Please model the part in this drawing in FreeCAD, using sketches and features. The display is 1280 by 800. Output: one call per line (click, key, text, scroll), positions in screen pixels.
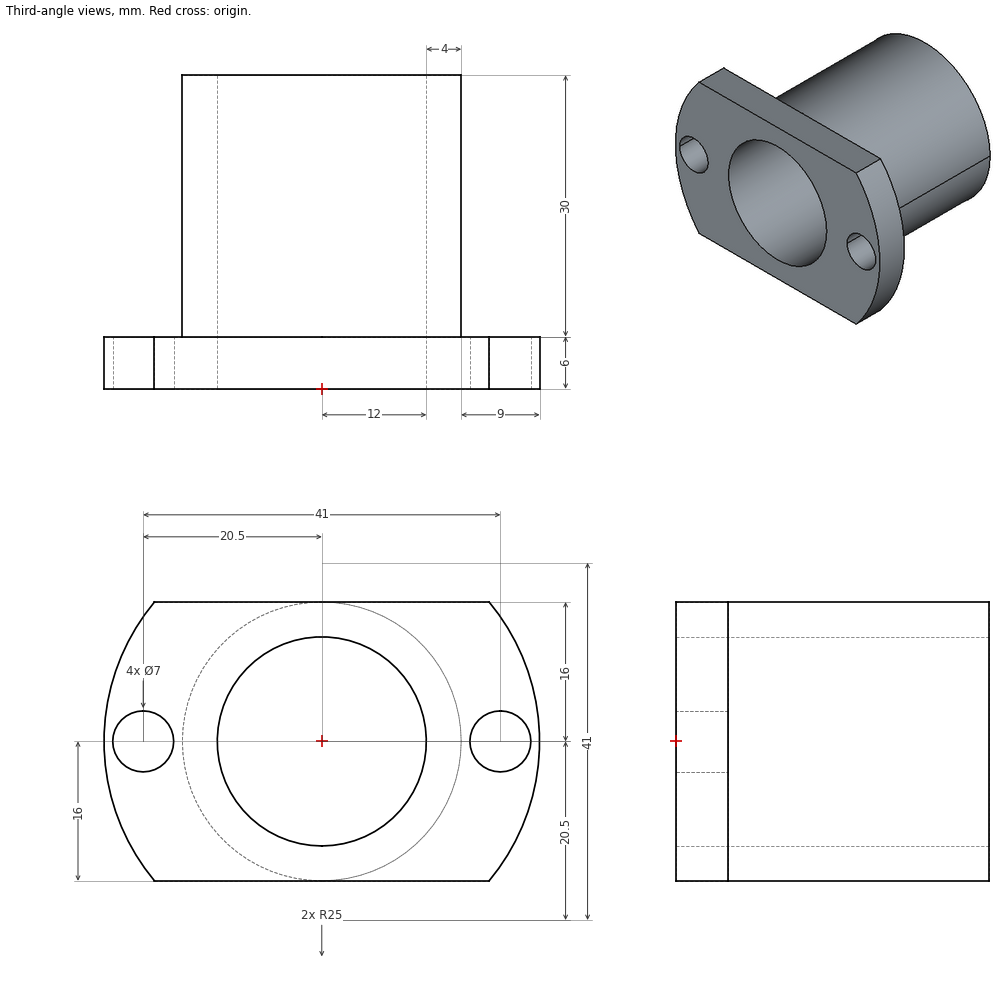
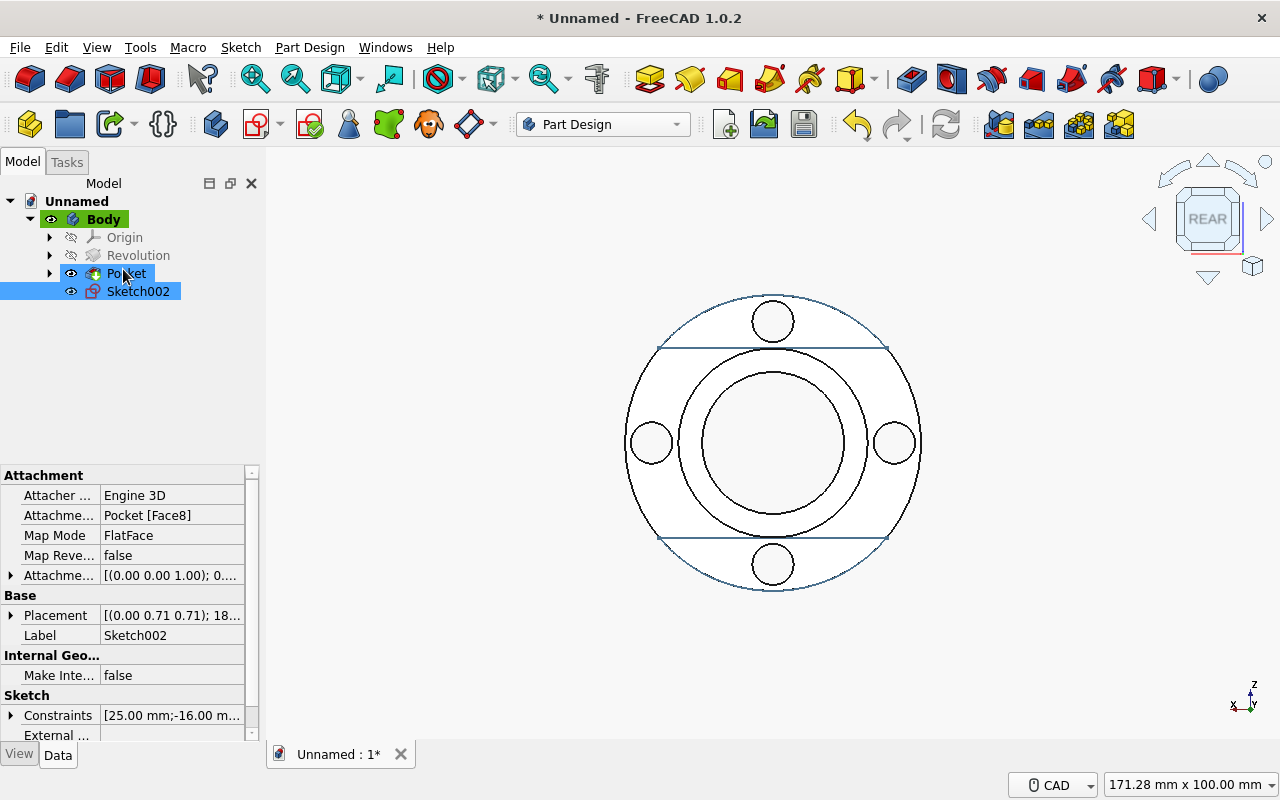
click(912, 80)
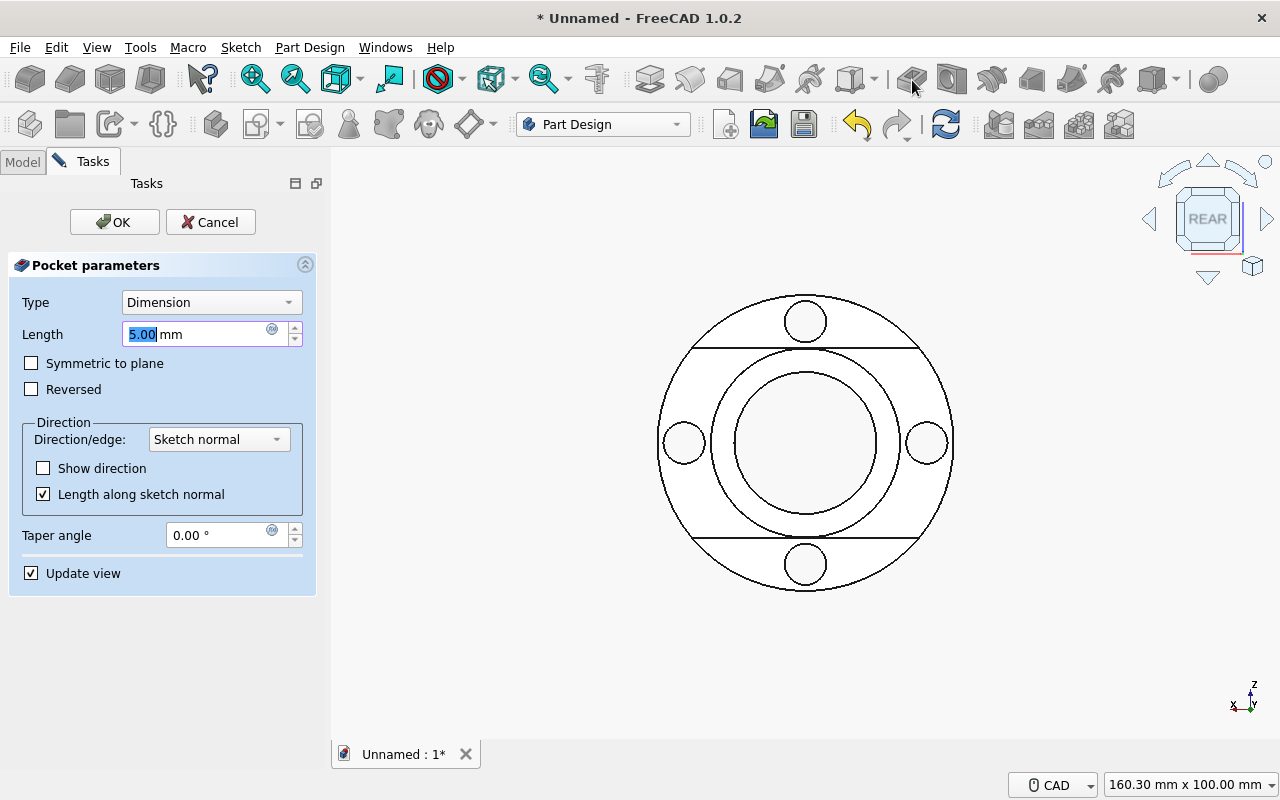
click(212, 302)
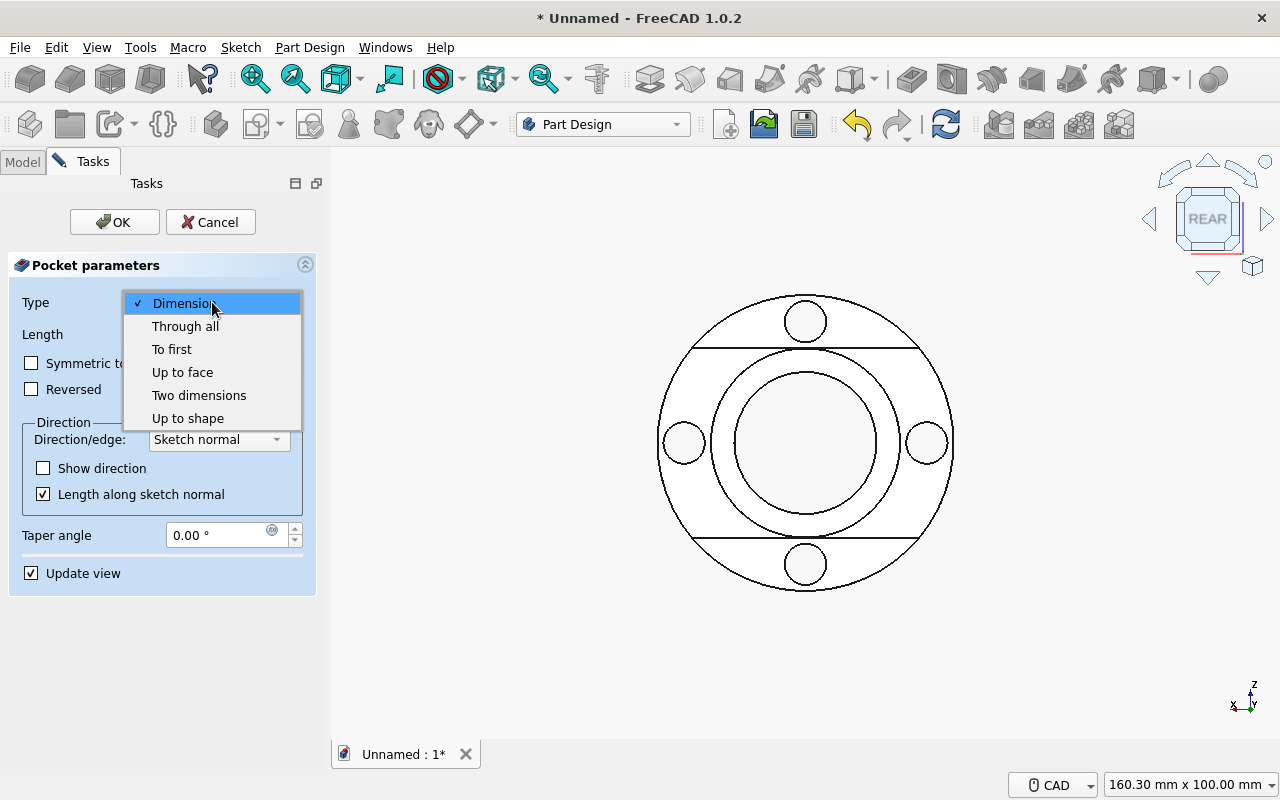
click(212, 326)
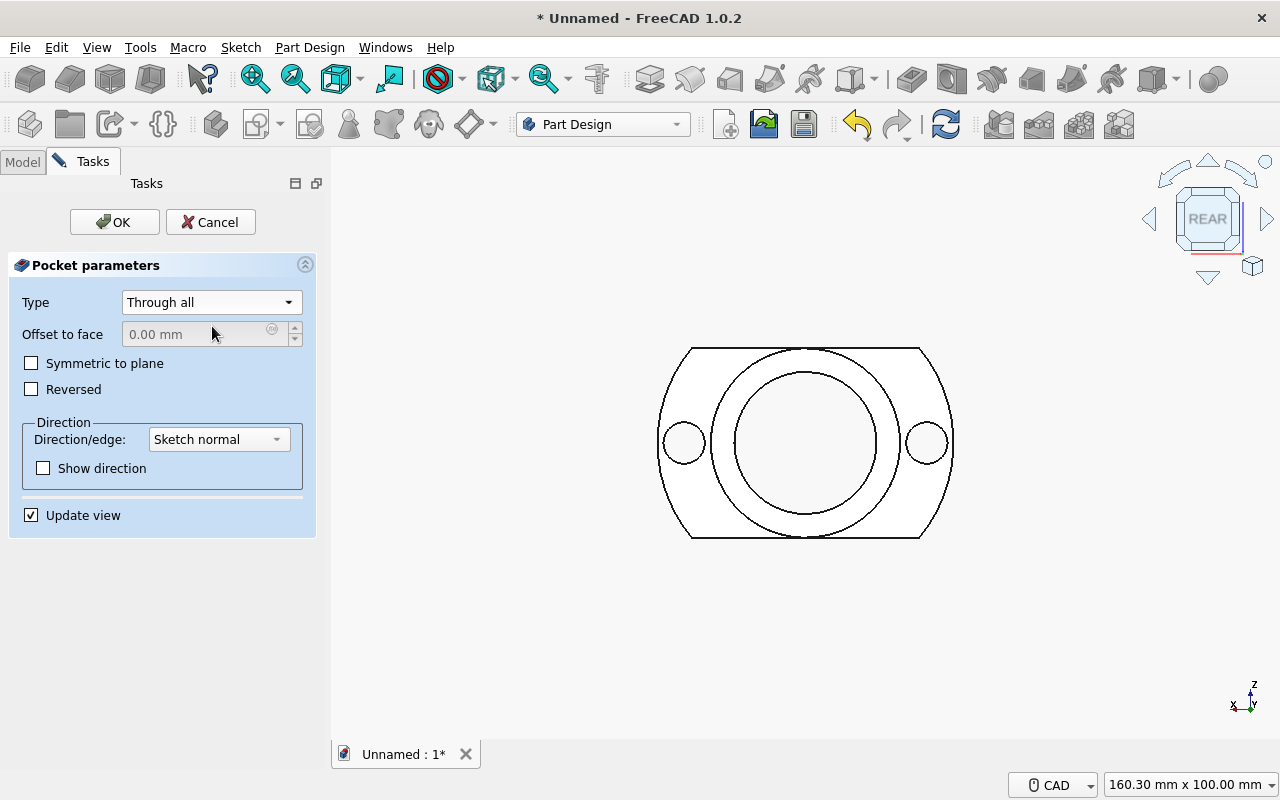
click(115, 222)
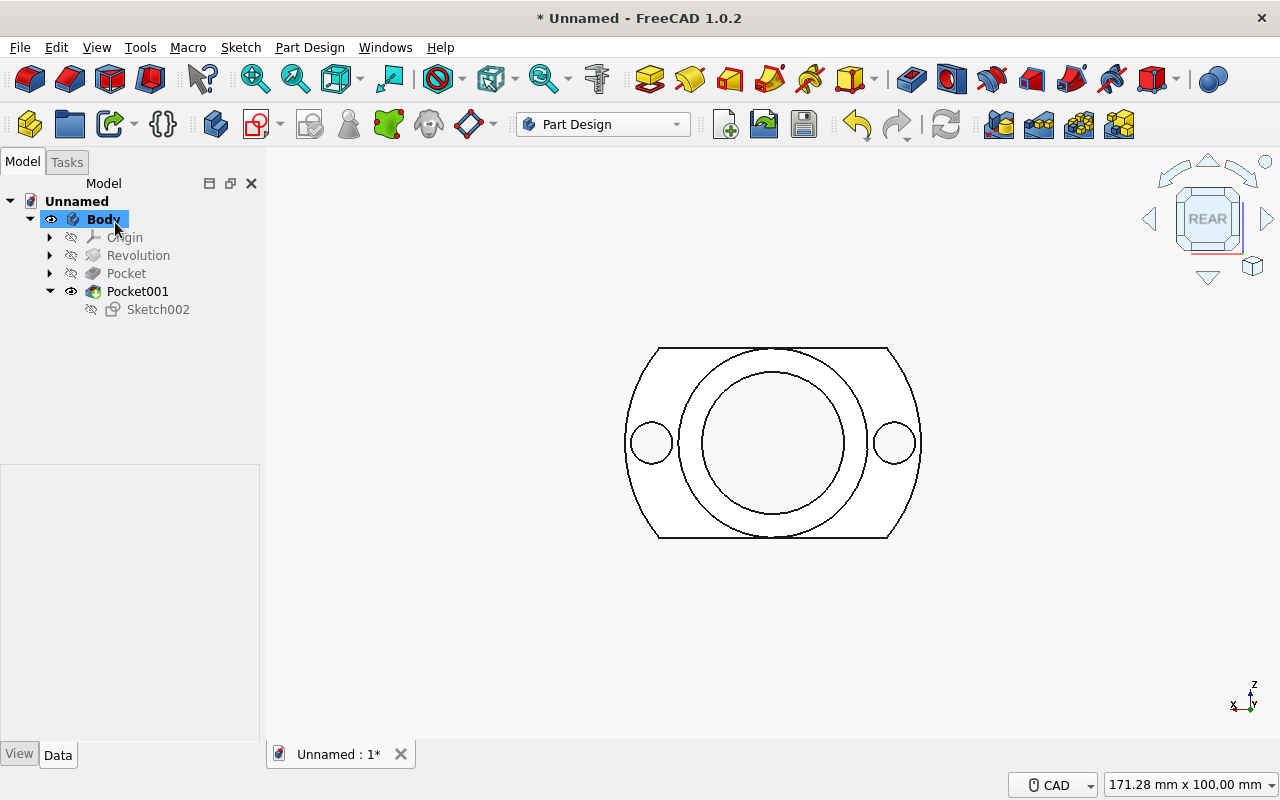
key(0)